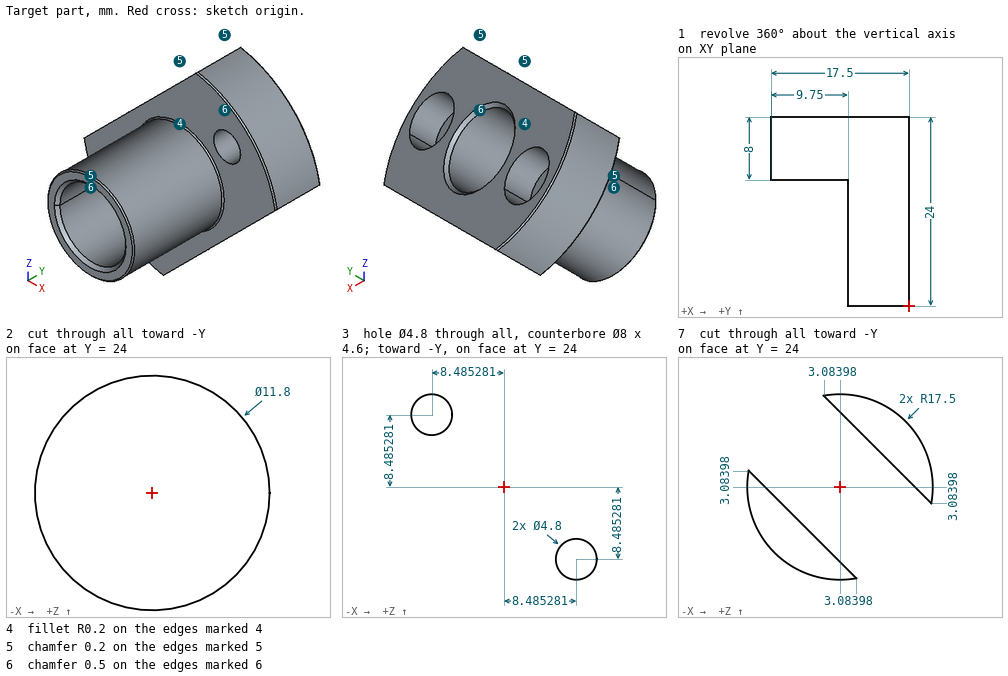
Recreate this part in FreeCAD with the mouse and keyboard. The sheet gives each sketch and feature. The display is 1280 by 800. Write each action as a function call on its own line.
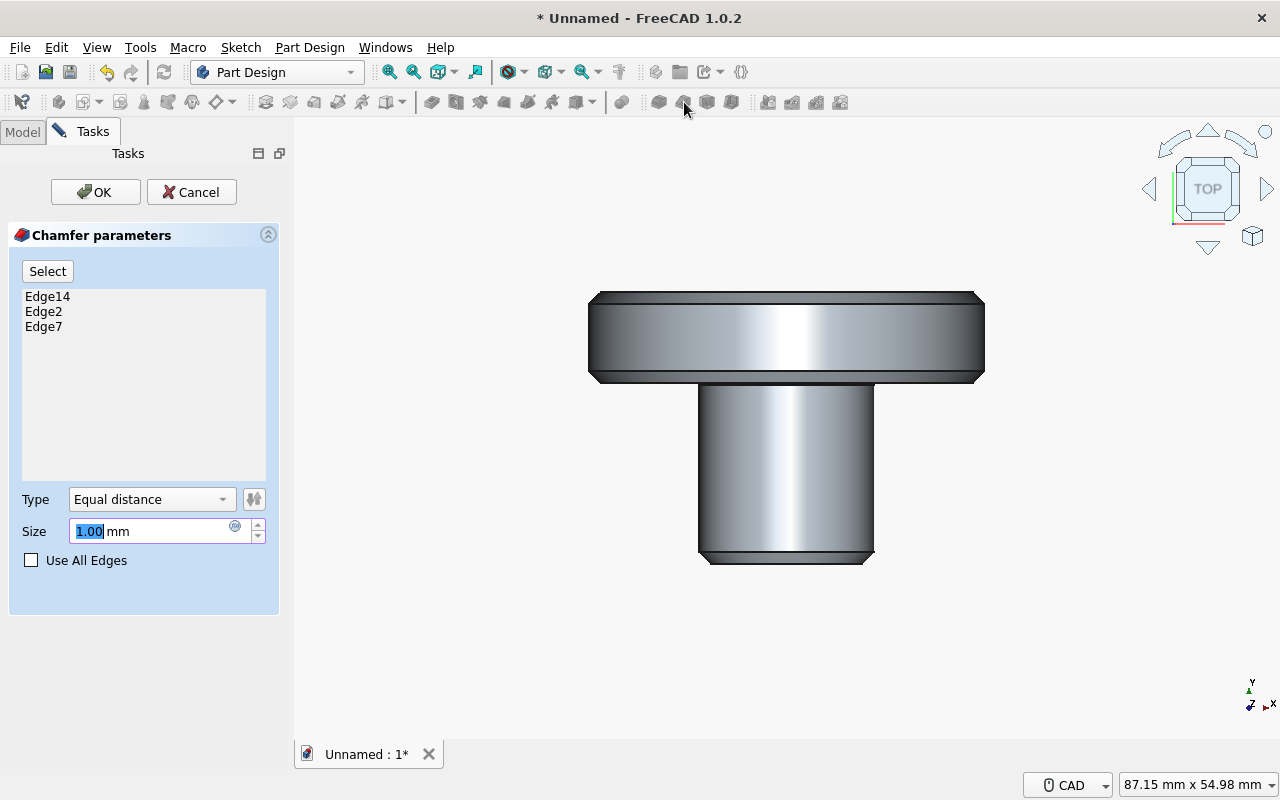
text(0.2)
key(Tab)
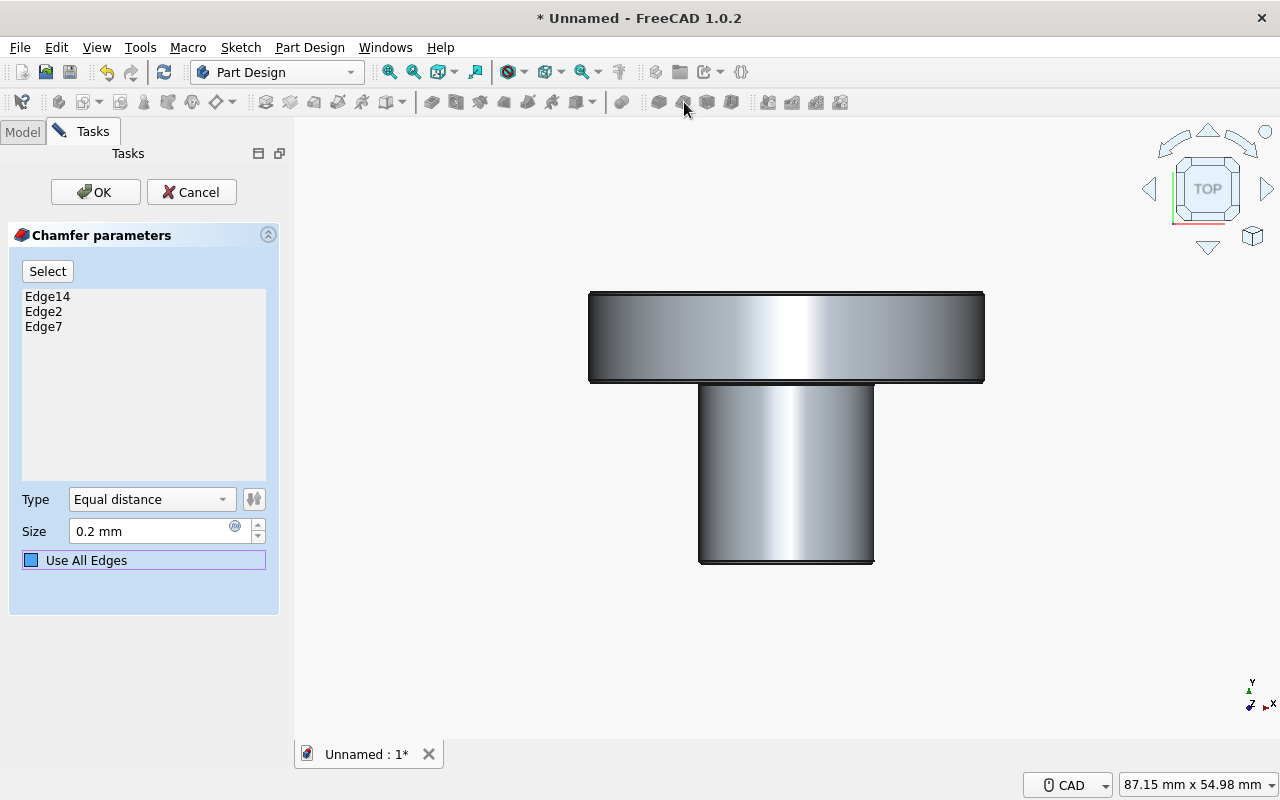
click(96, 192)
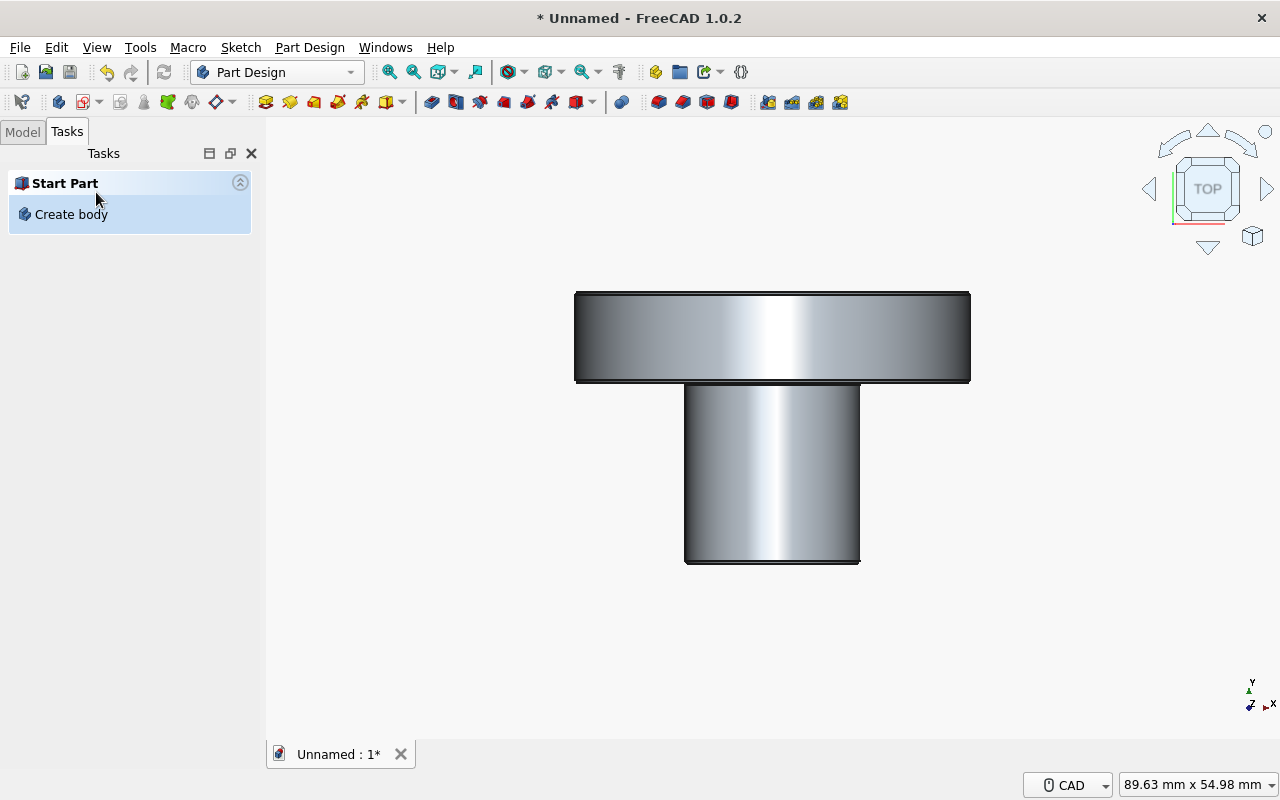
key(v)
key(f)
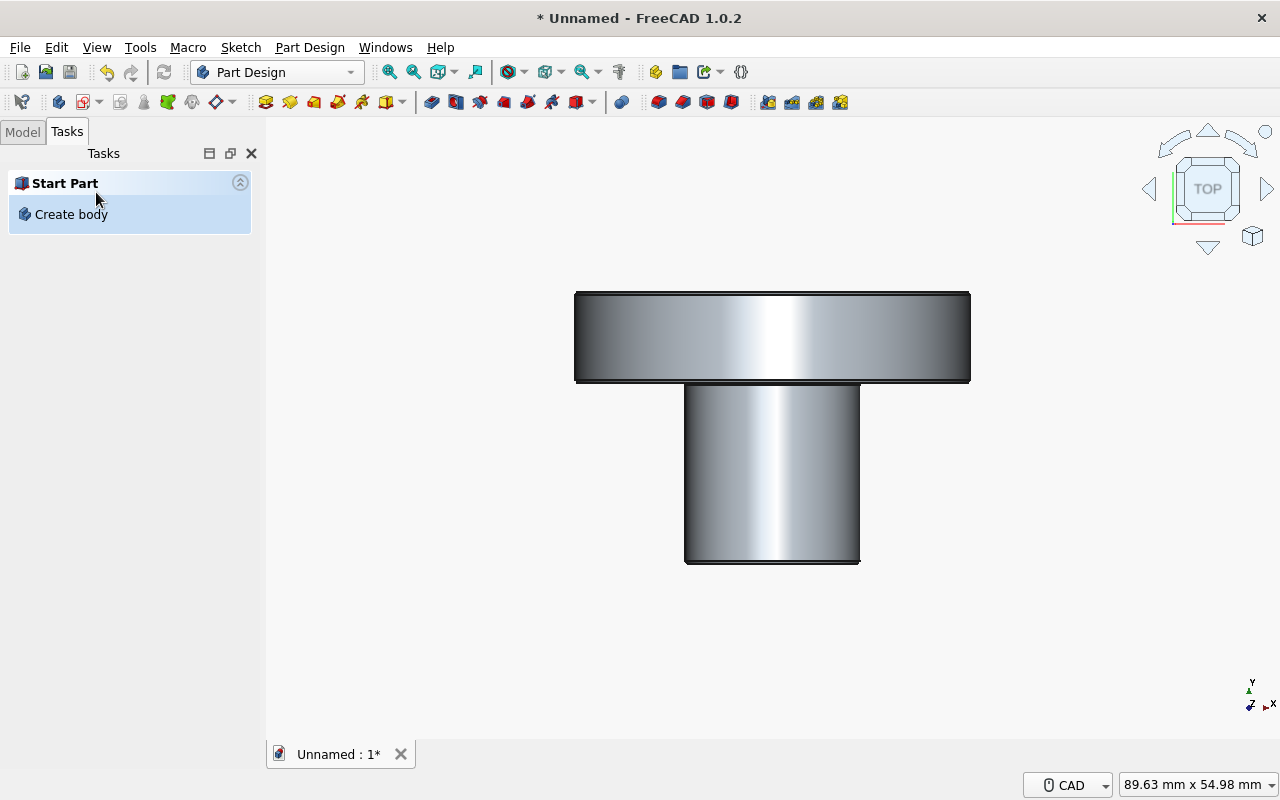
key(0)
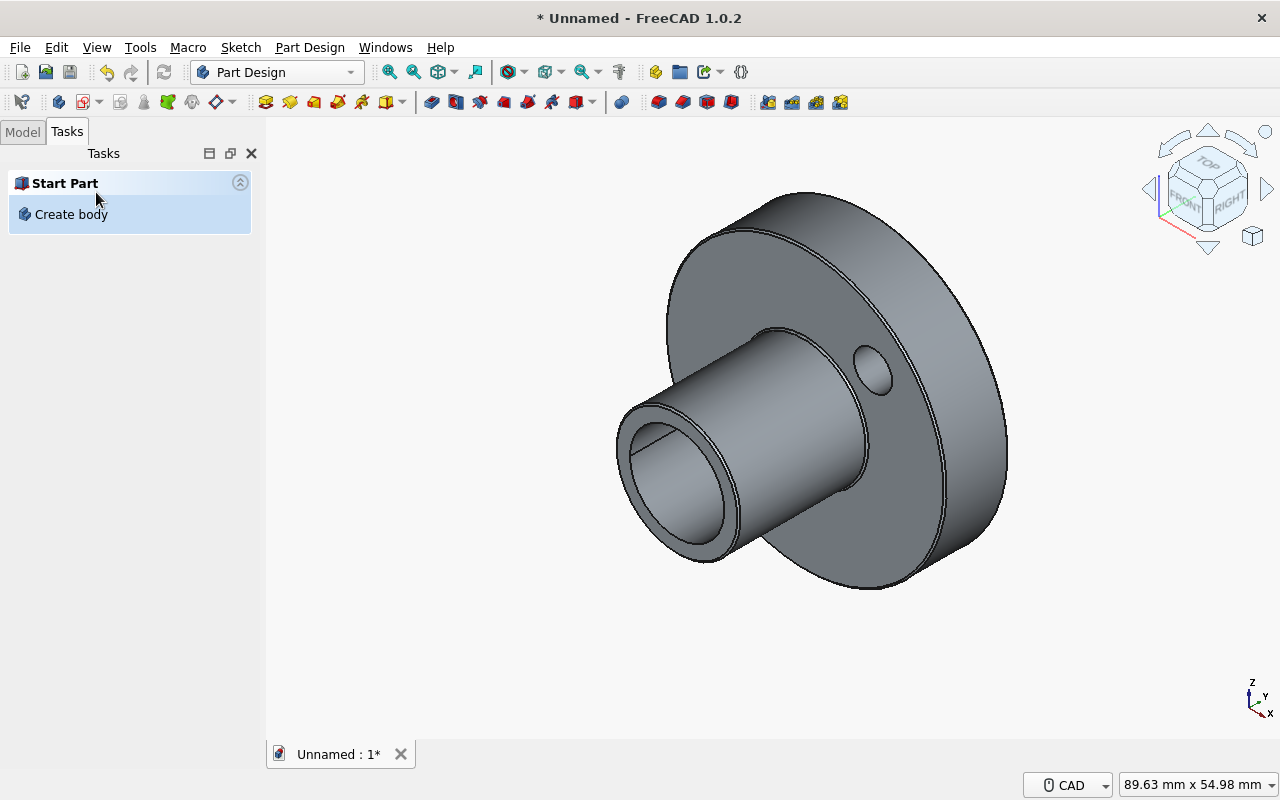
click(692, 543)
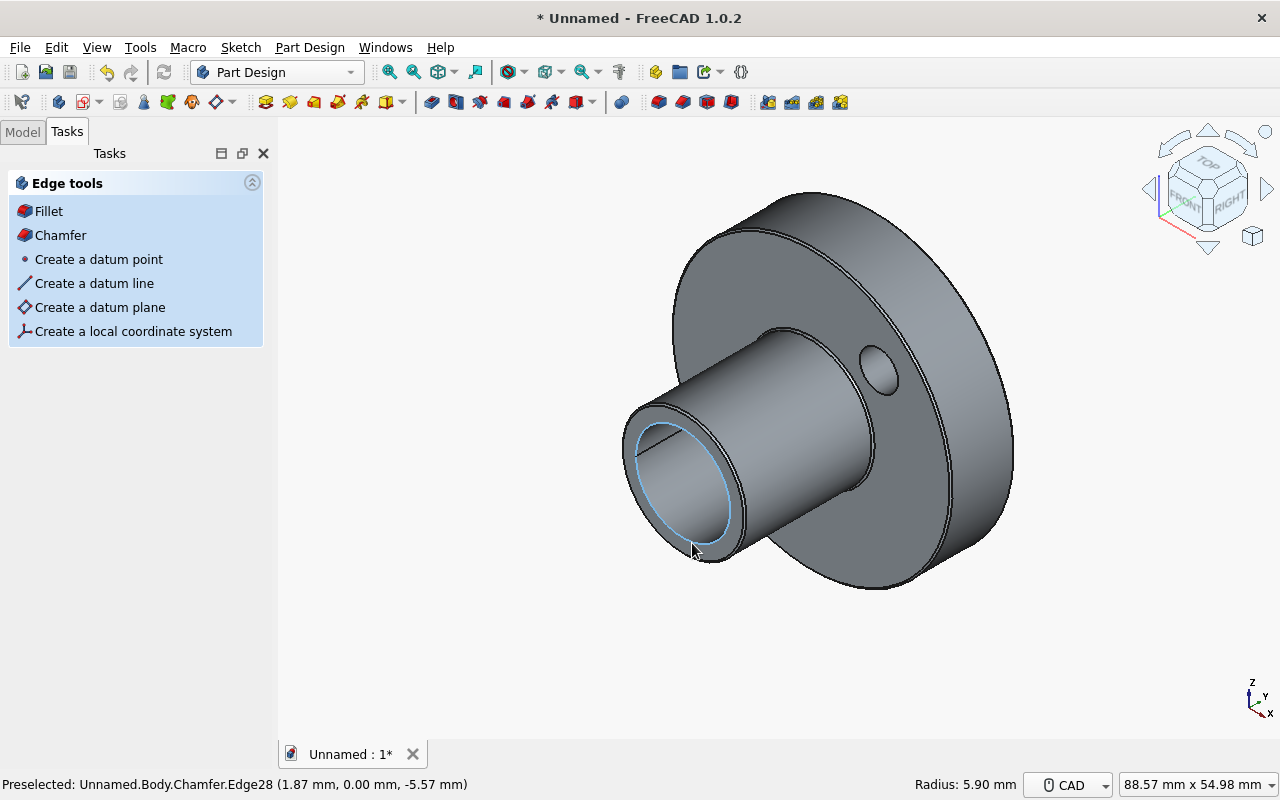
key(2)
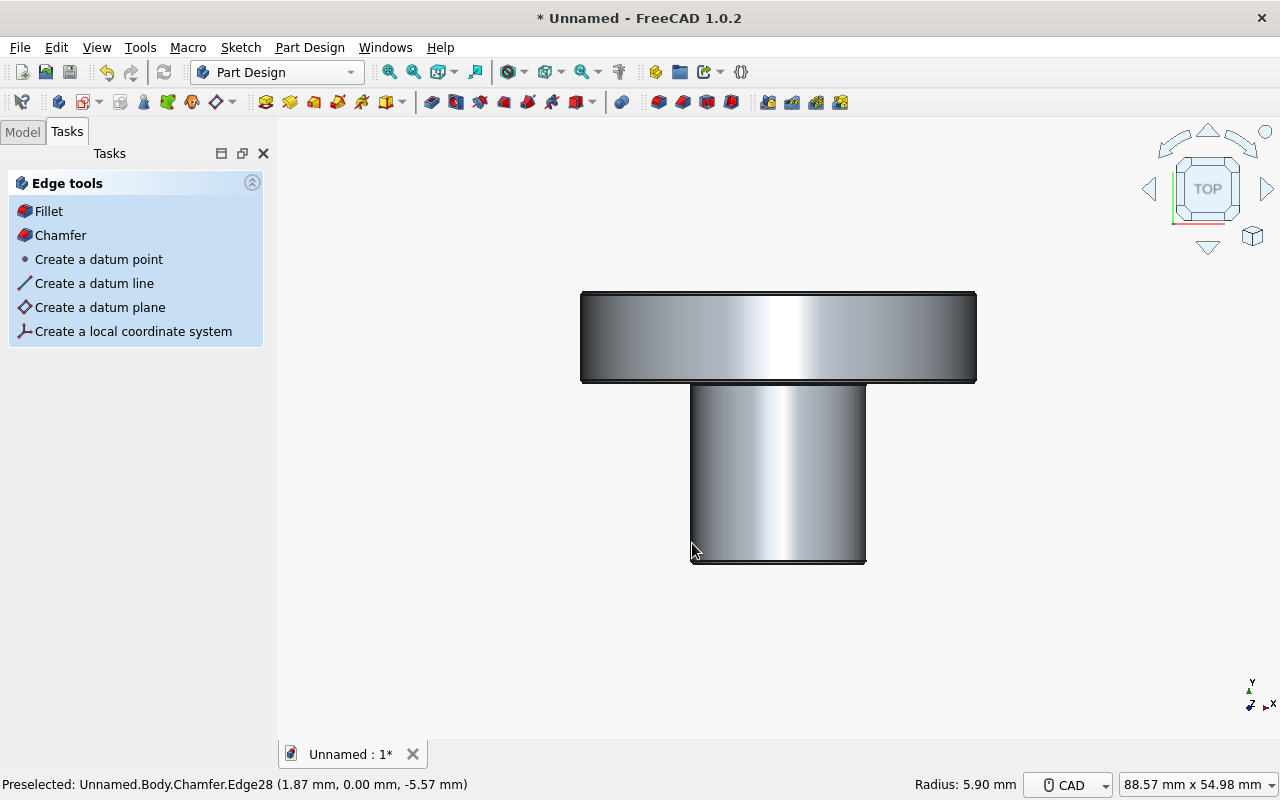
click(390, 72)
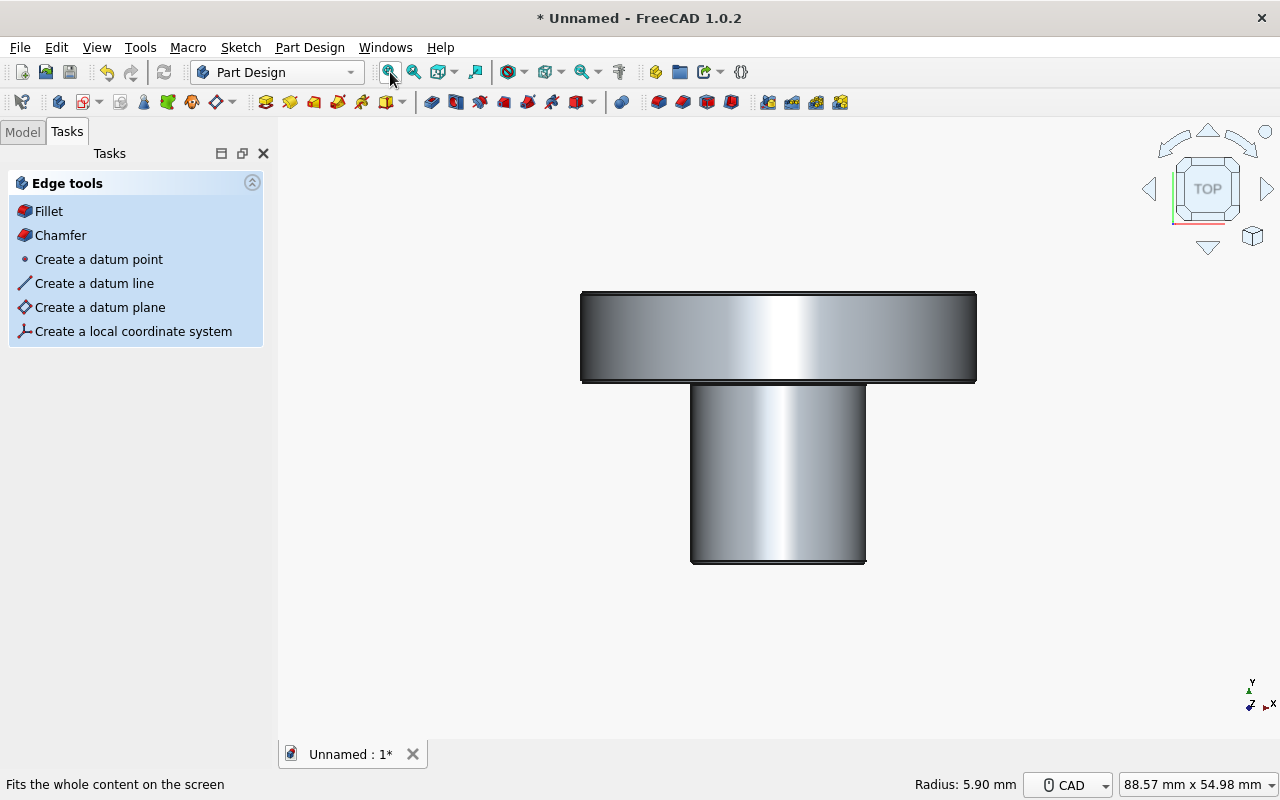
key(1)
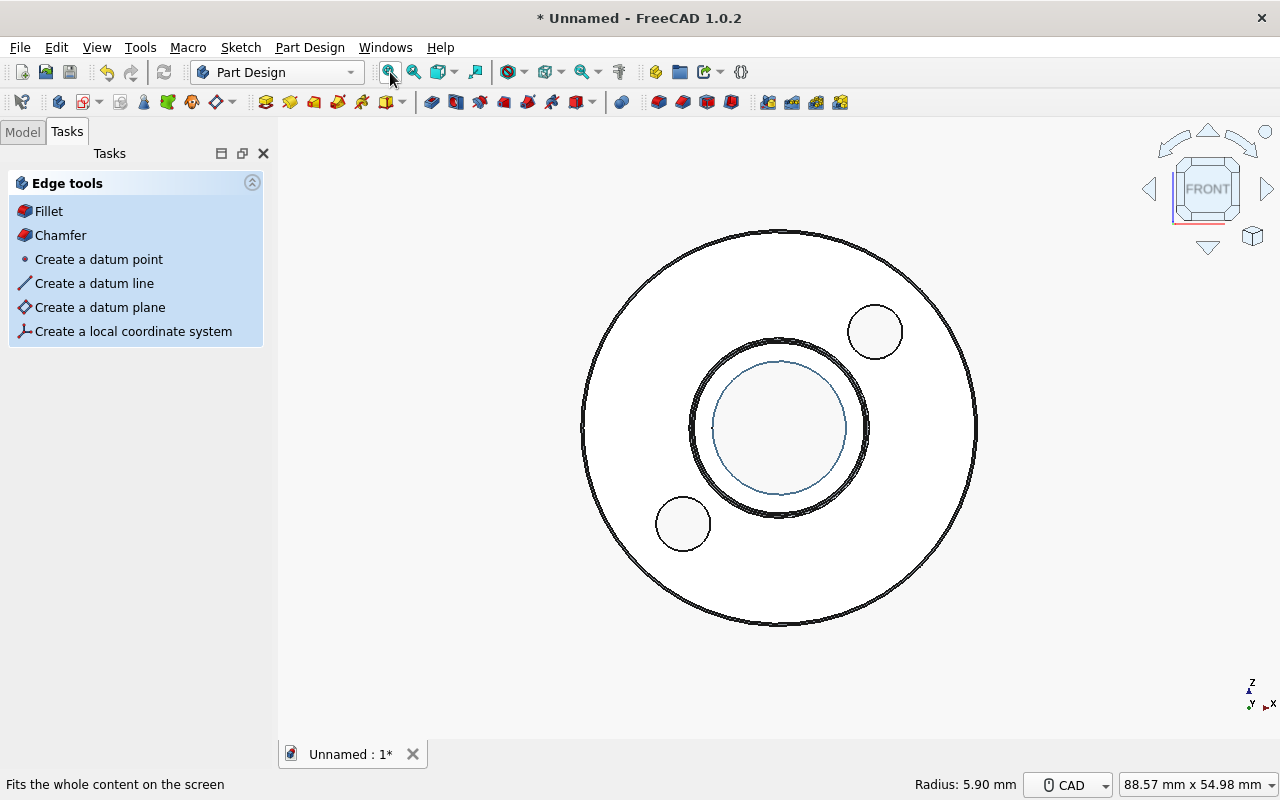
key(3)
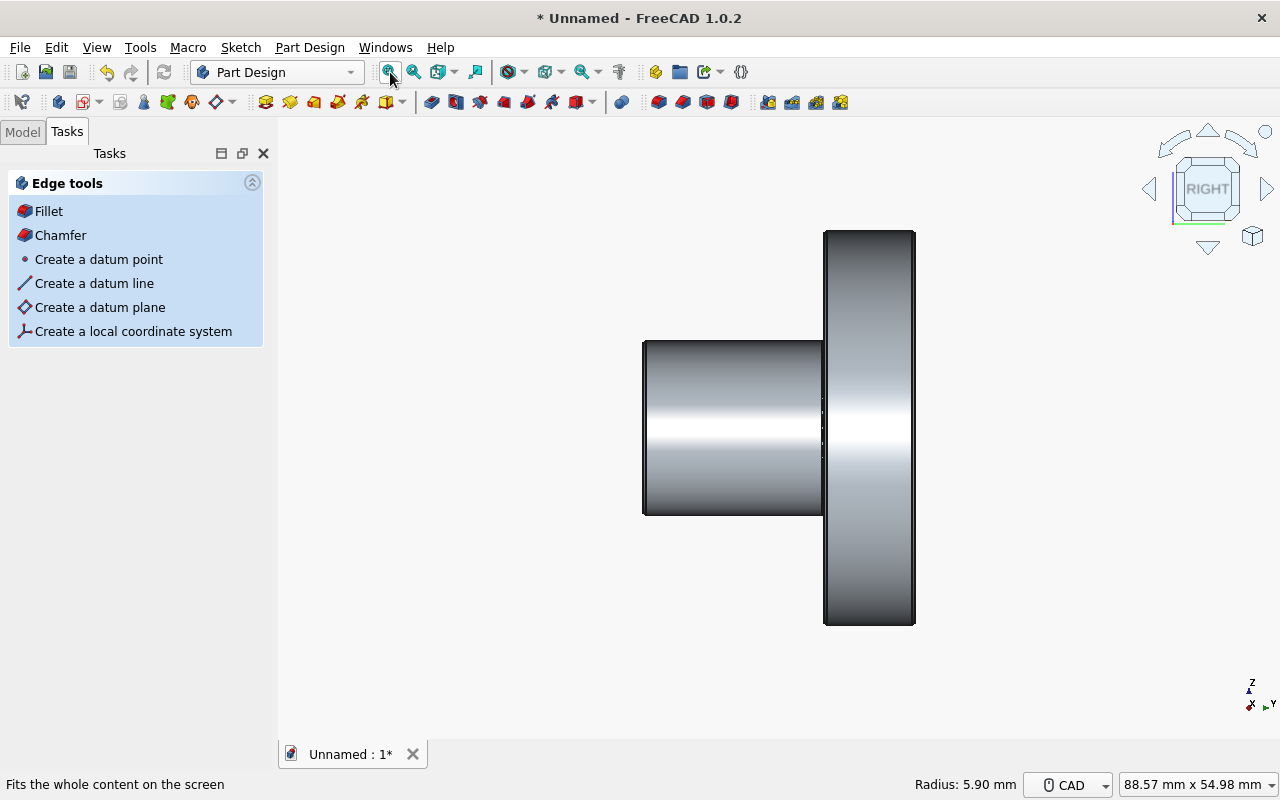
key(5)